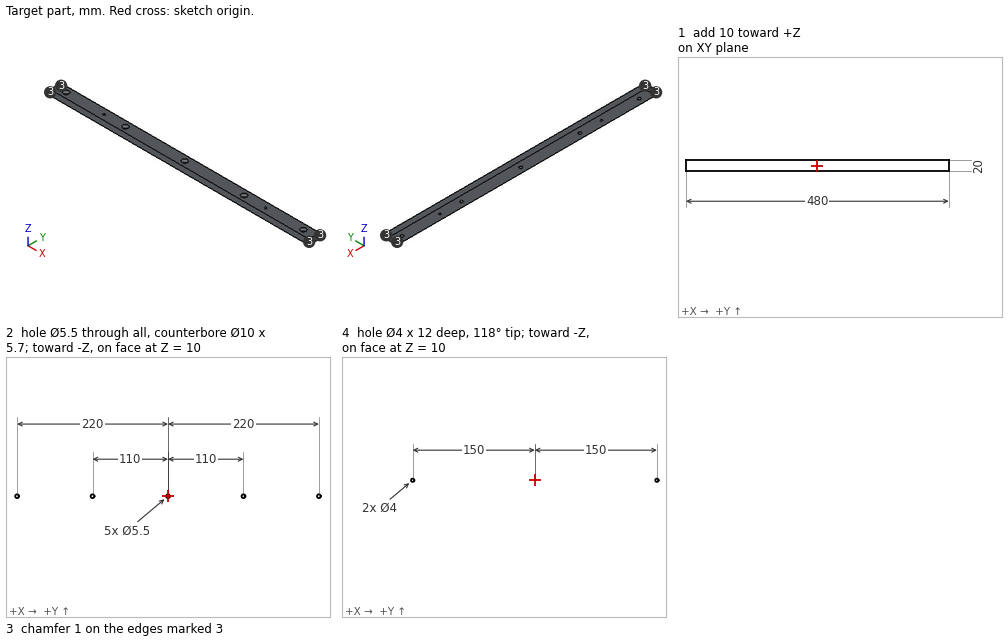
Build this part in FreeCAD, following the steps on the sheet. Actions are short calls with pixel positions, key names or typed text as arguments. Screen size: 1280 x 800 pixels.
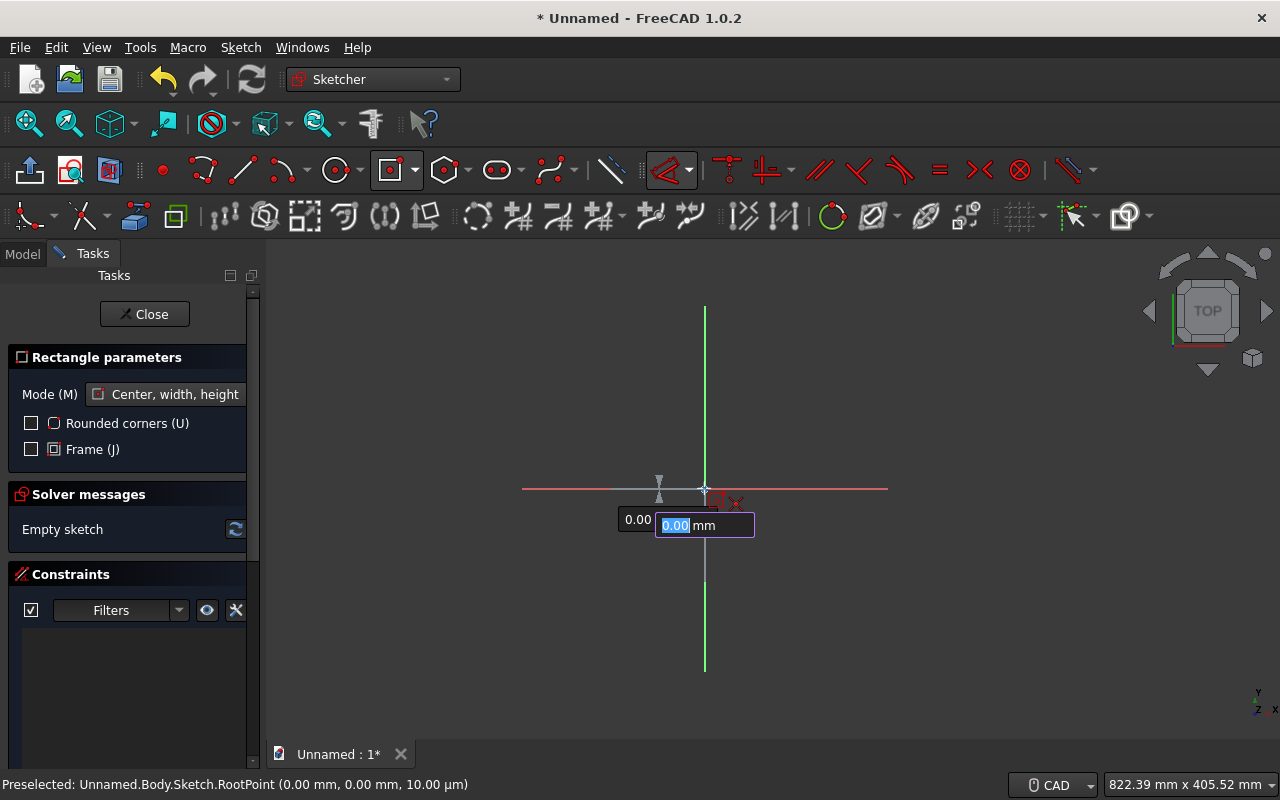
scroll(1001, 477, up, 2)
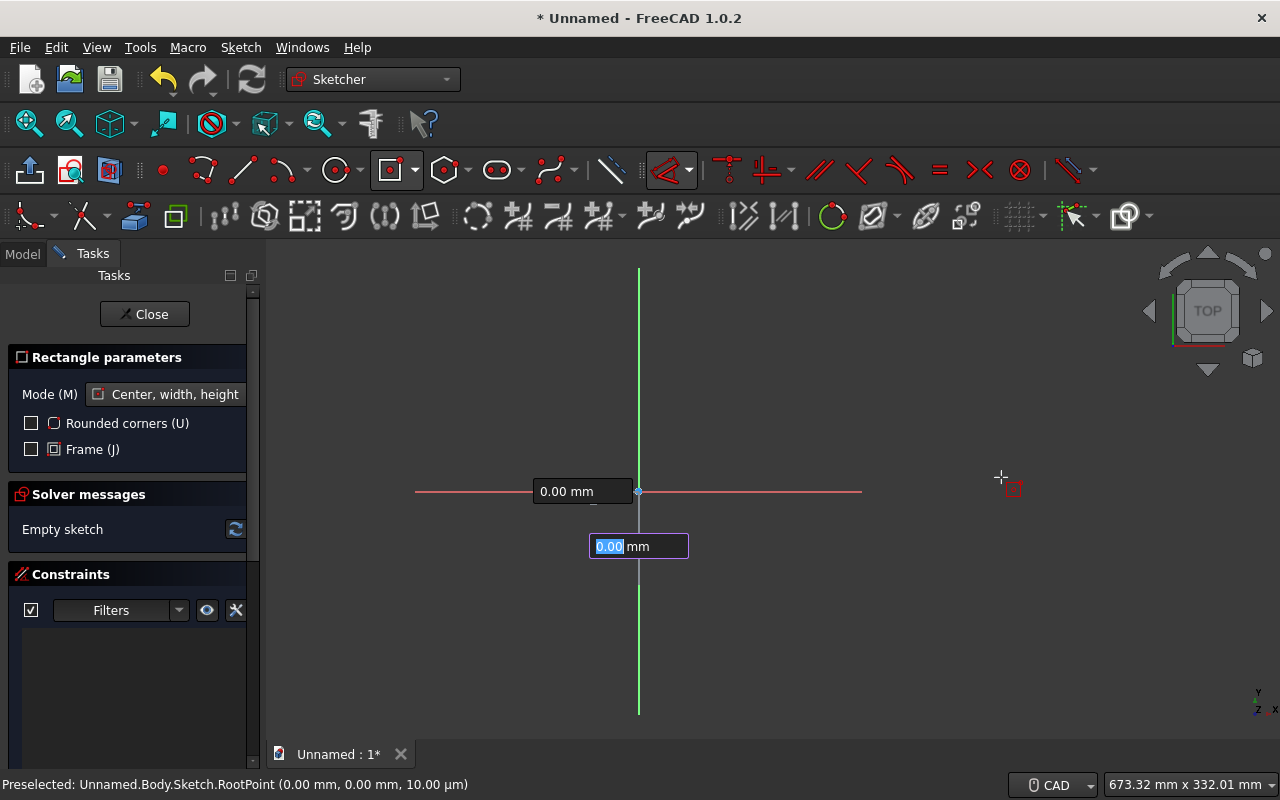
click(1000, 476)
key(Escape)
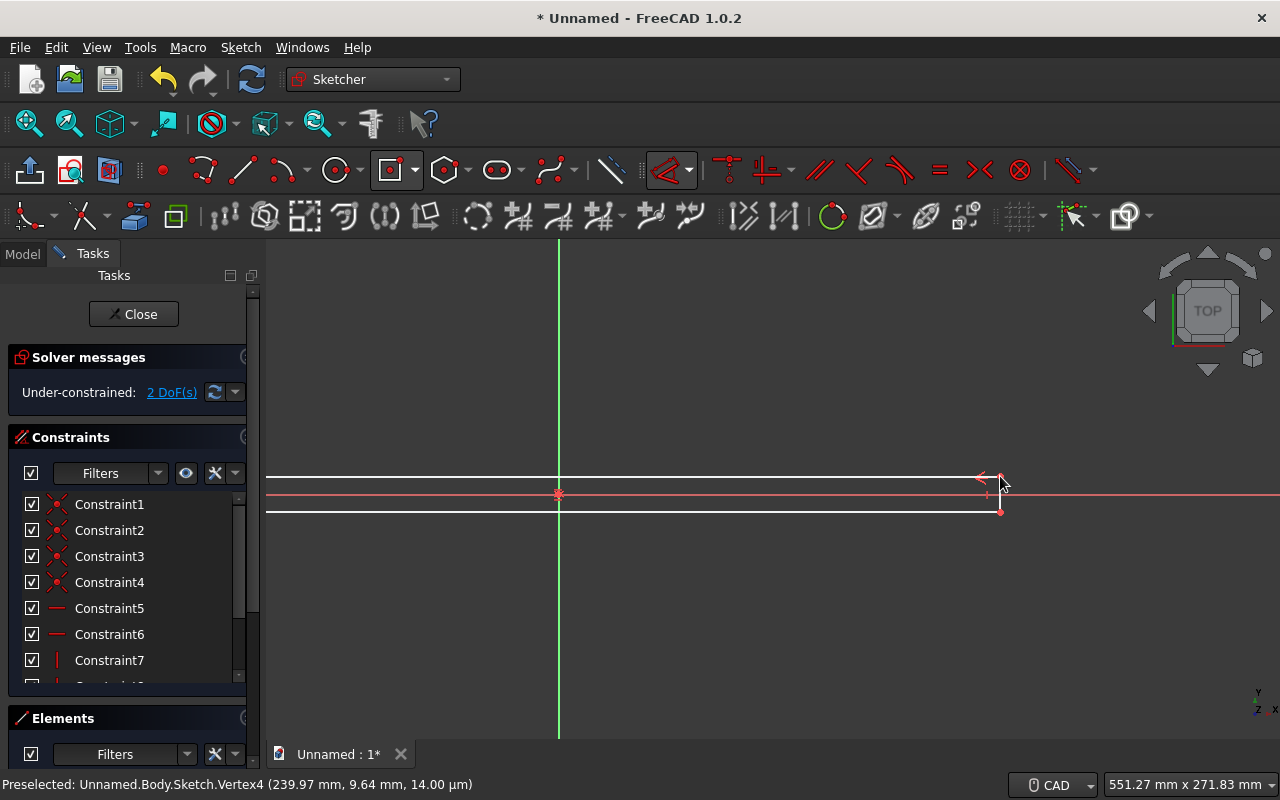
click(666, 170)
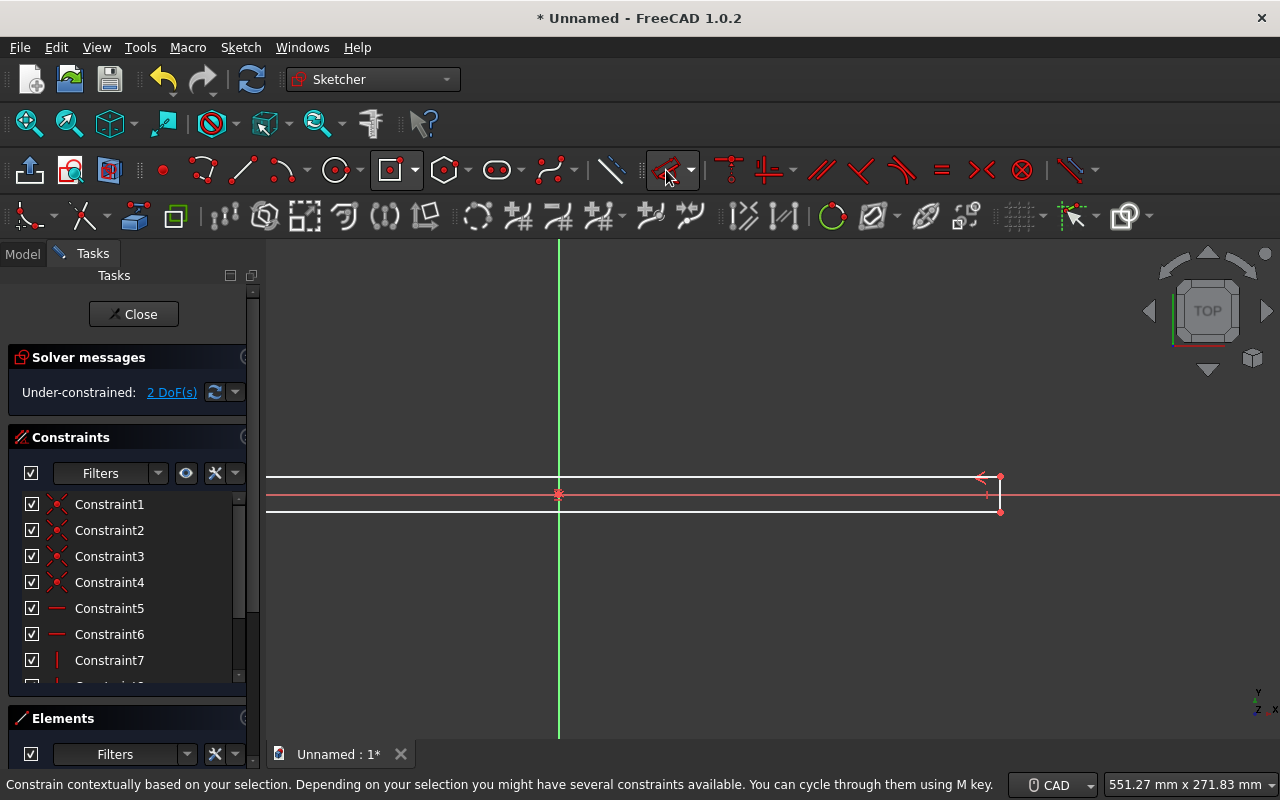
click(1000, 498)
click(1034, 487)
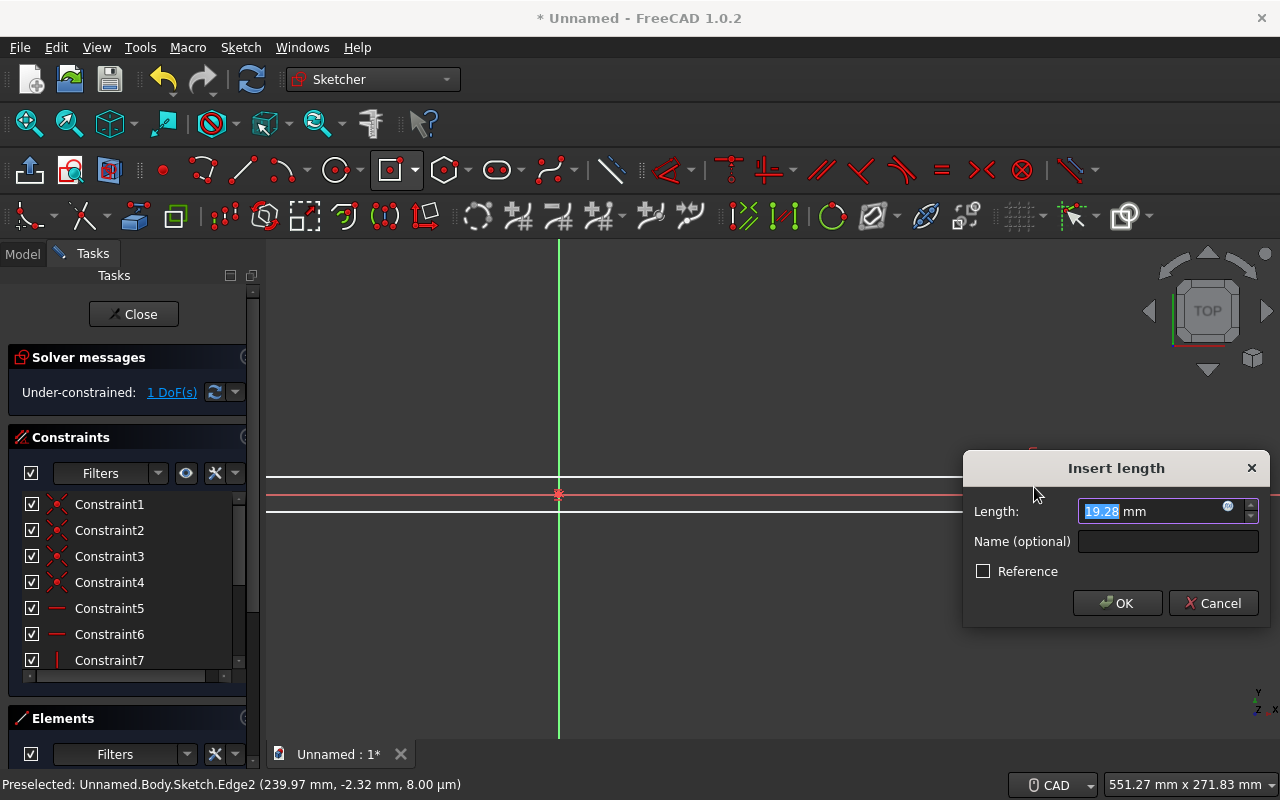
text(20)
key(Return)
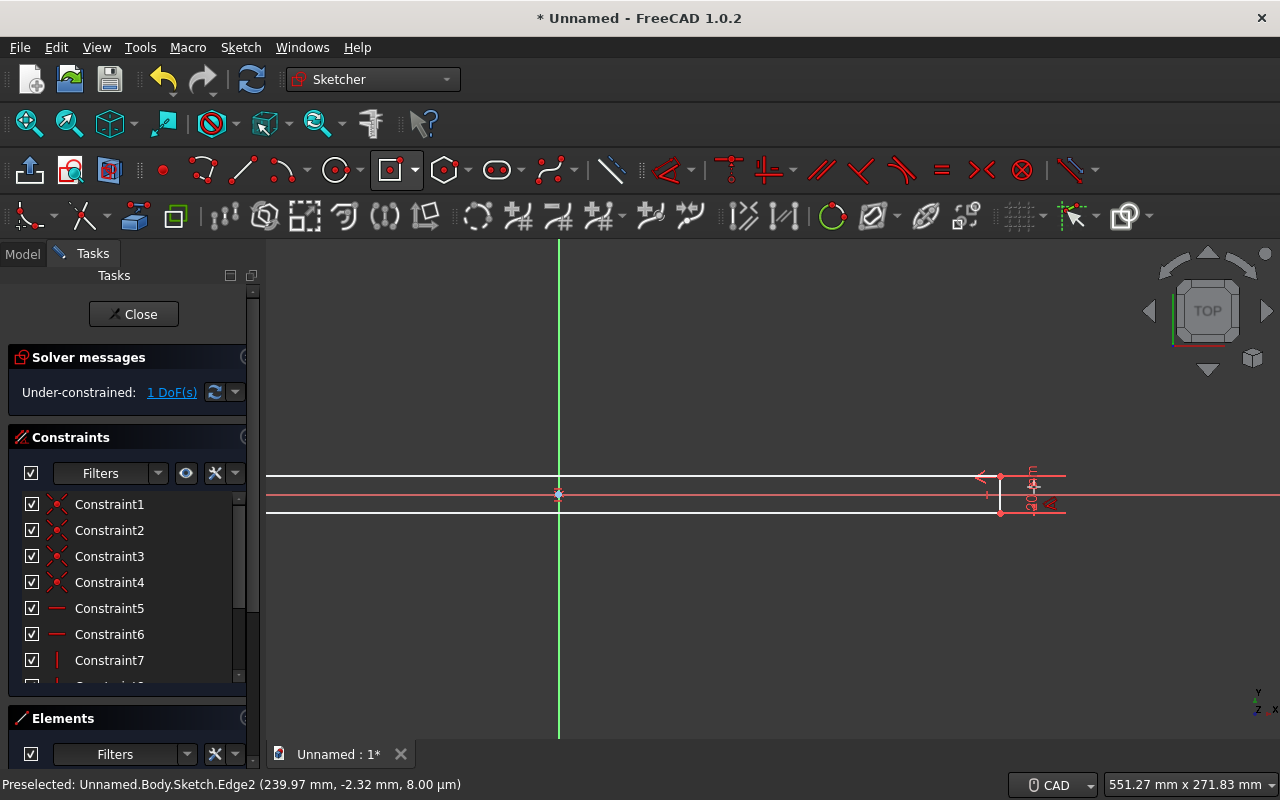
click(382, 513)
click(647, 547)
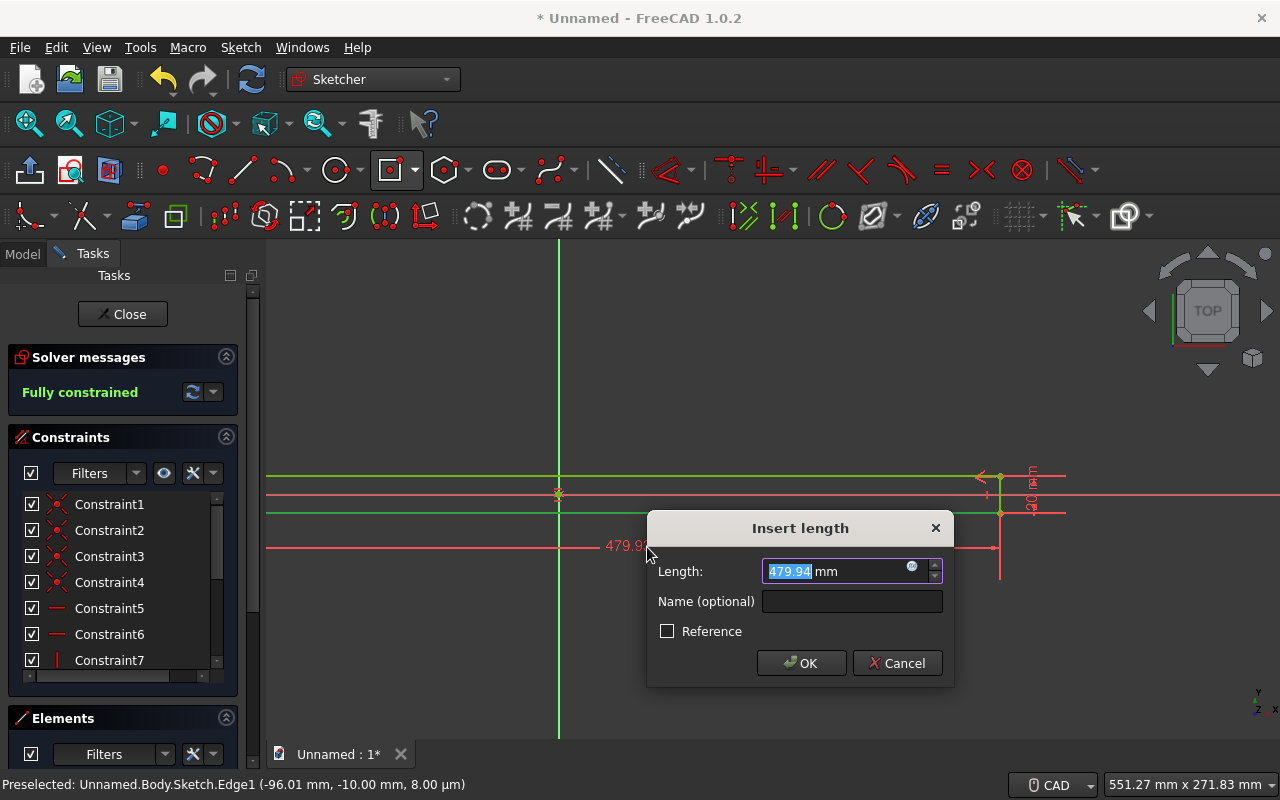
text(480)
key(Return)
key(Escape)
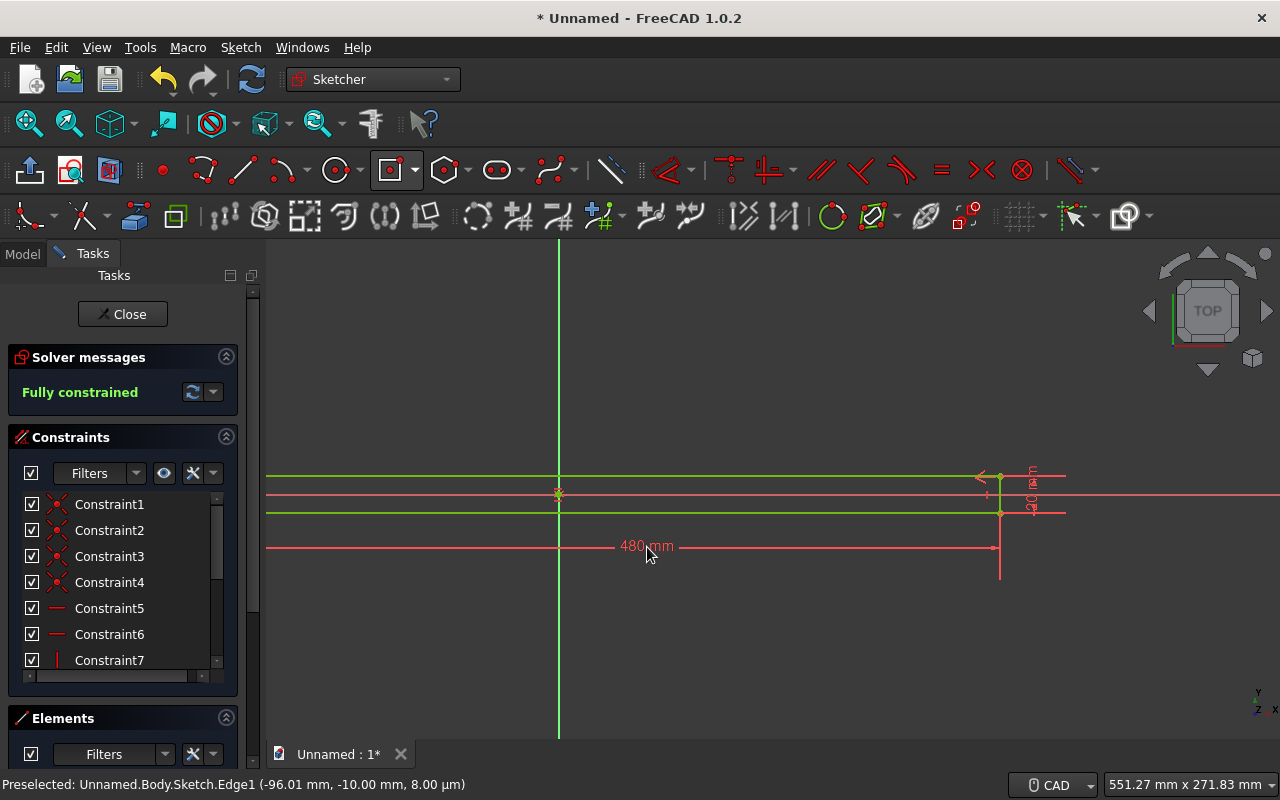
click(123, 314)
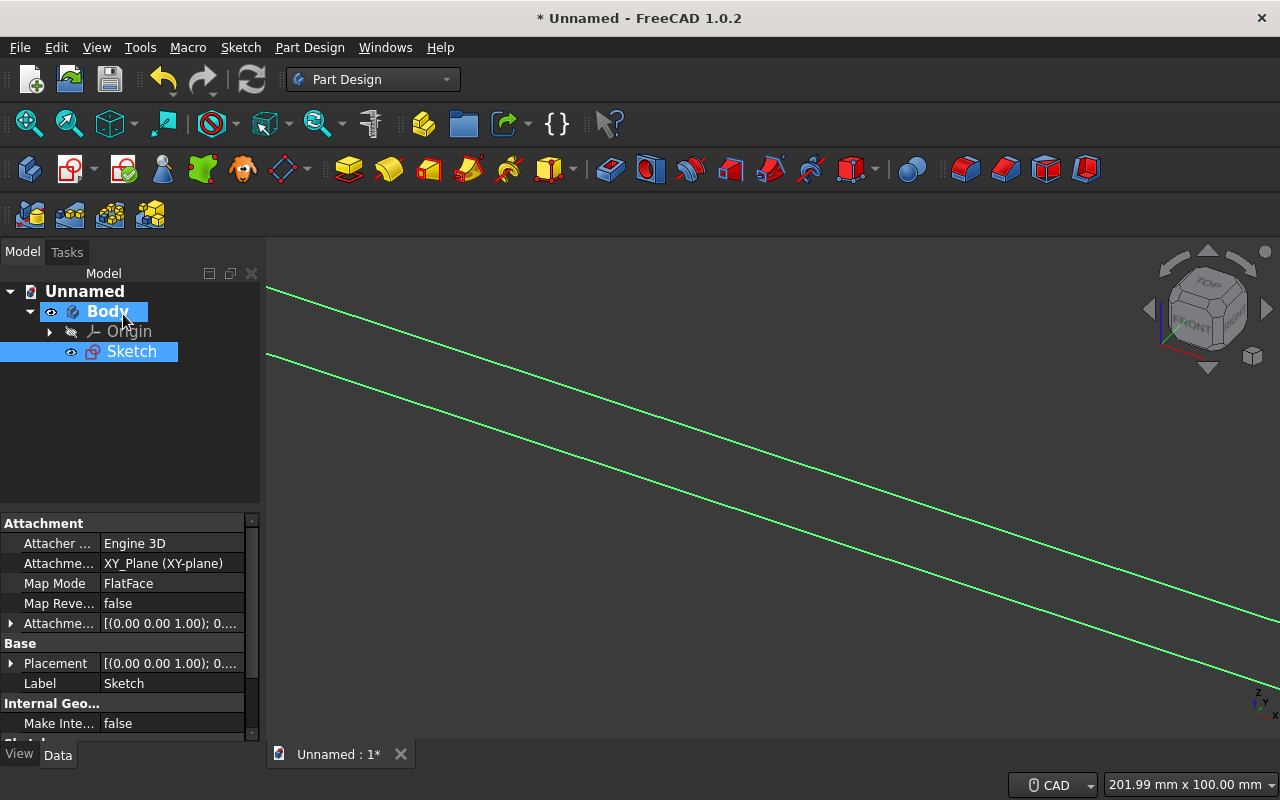
click(350, 170)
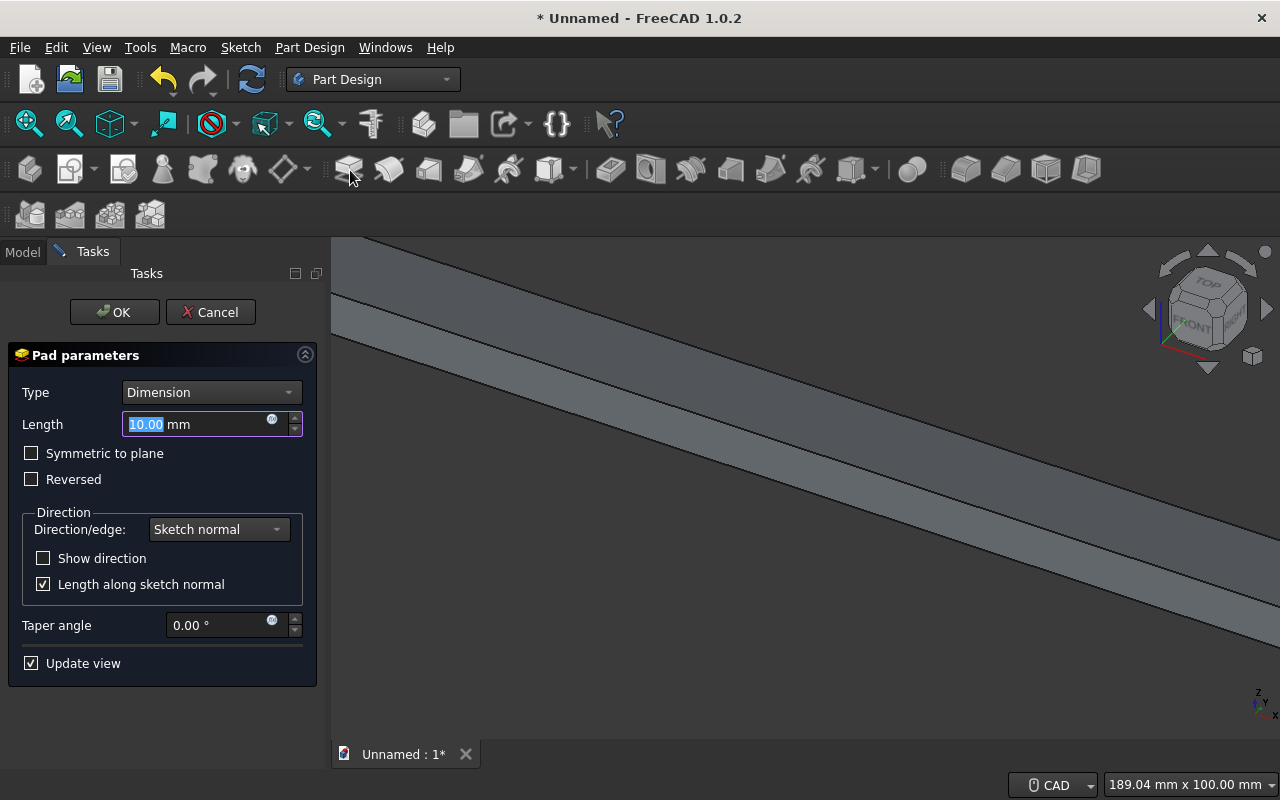
text(10)
key(Tab)